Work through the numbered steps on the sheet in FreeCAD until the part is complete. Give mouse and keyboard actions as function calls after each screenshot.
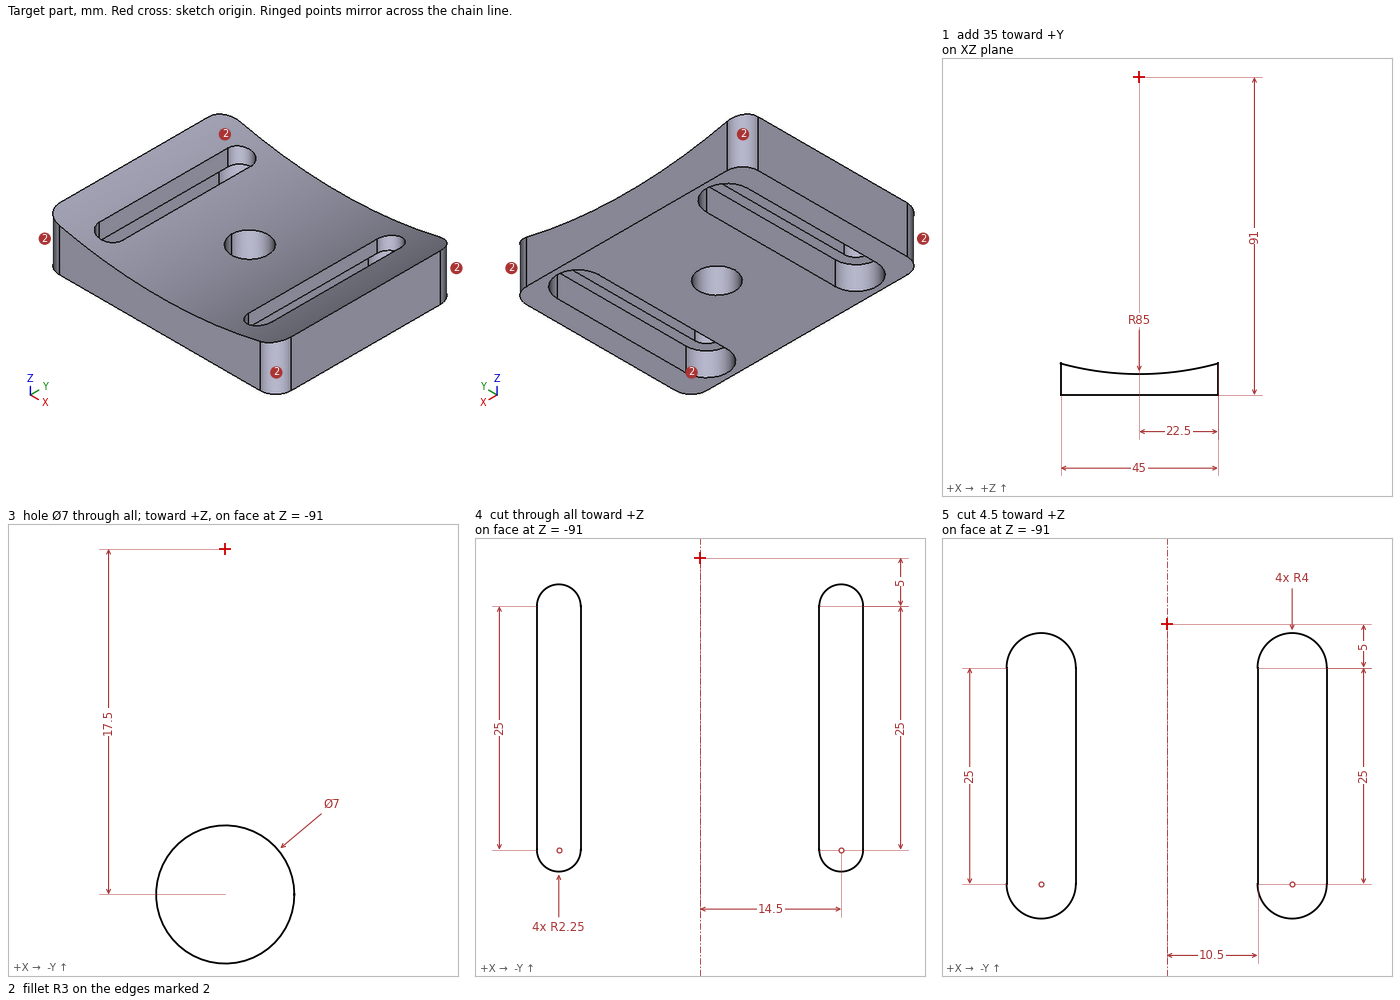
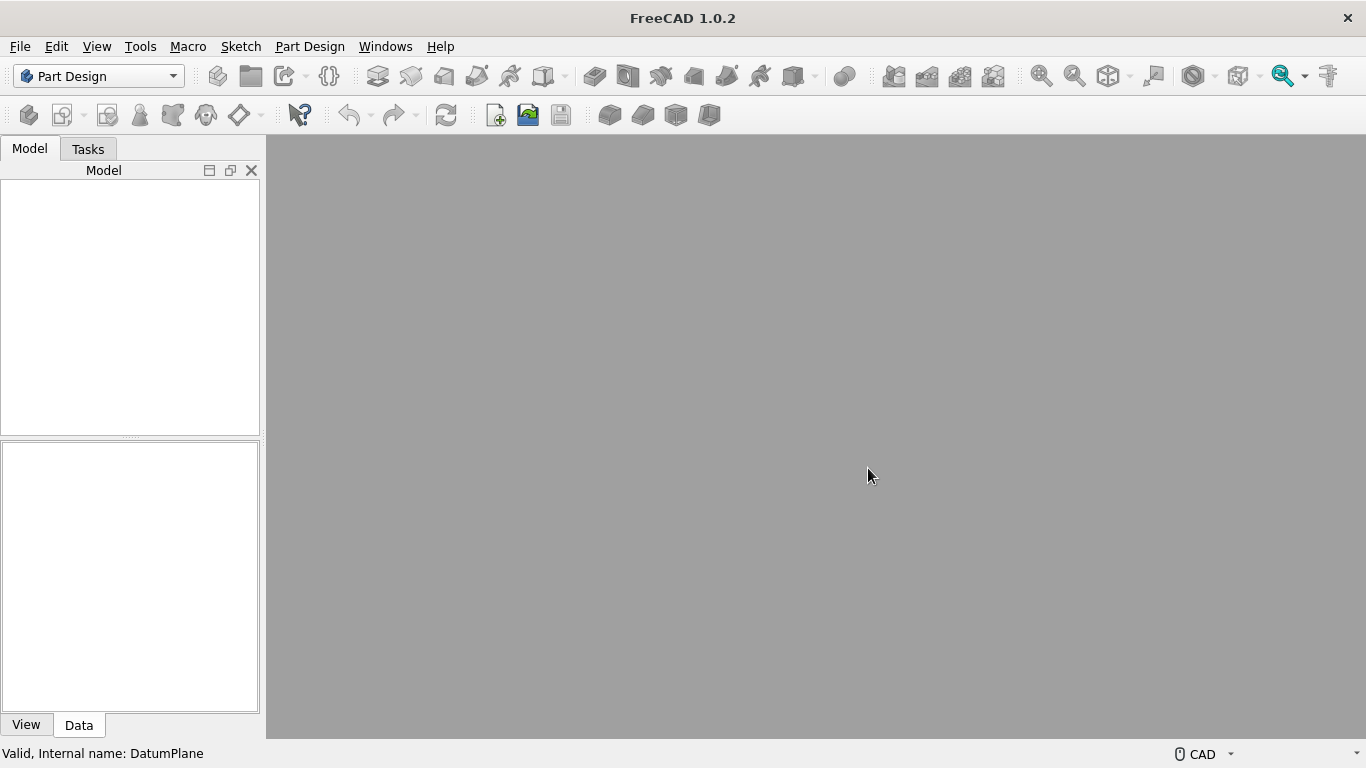
click(495, 116)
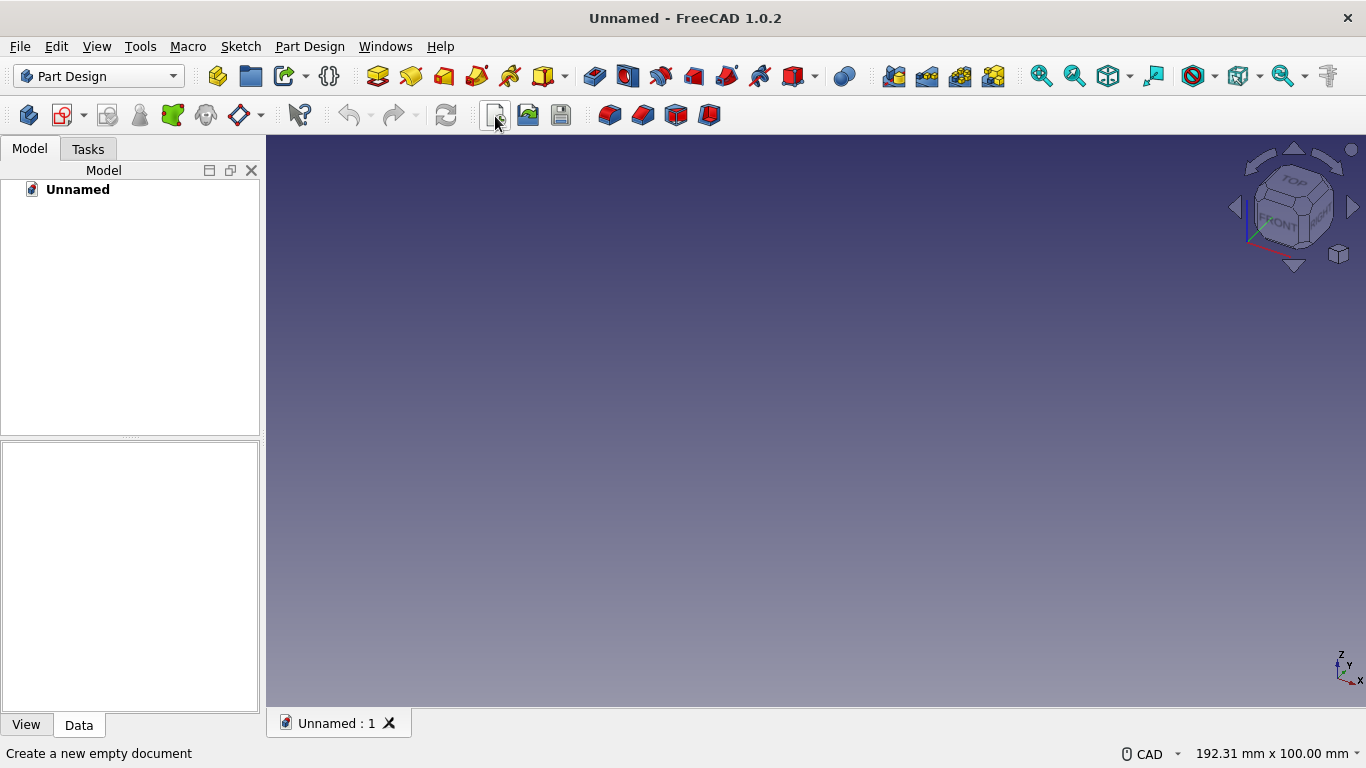
click(62, 116)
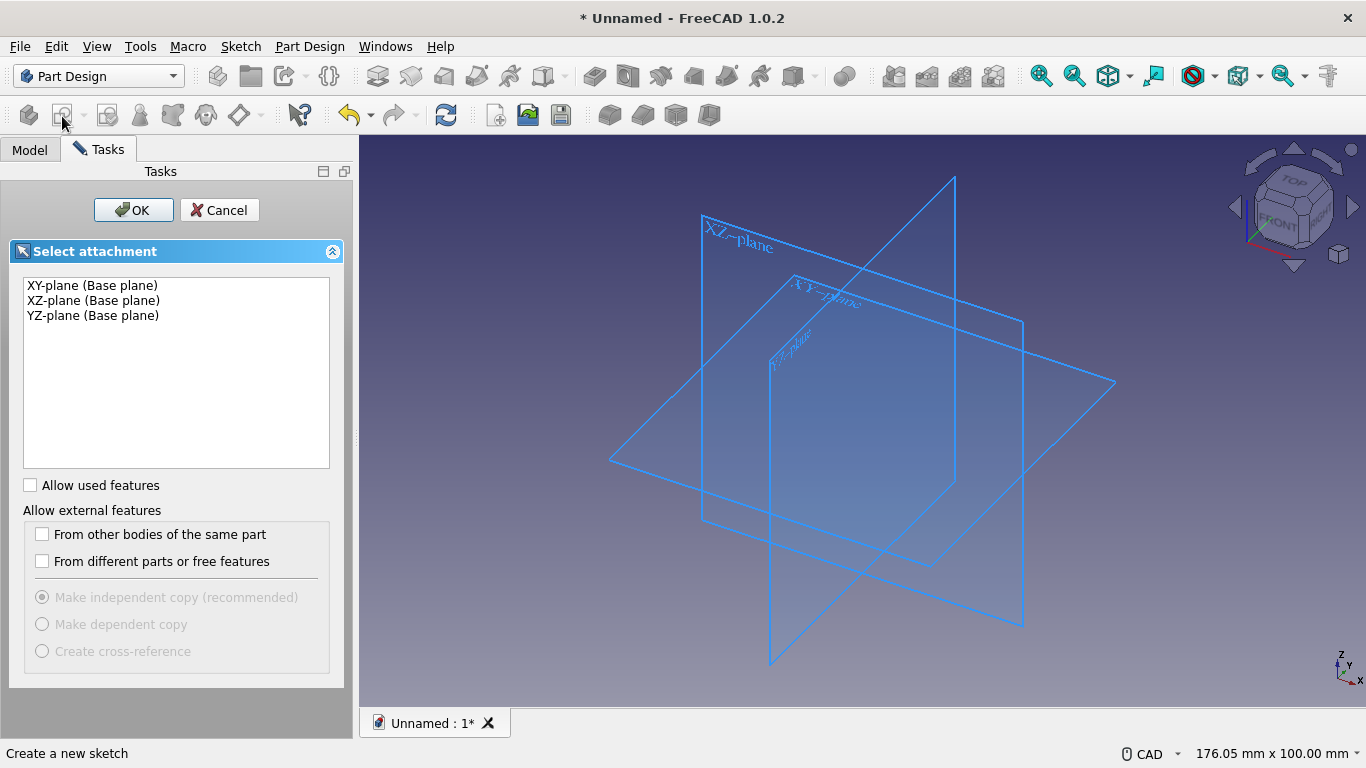
click(84, 300)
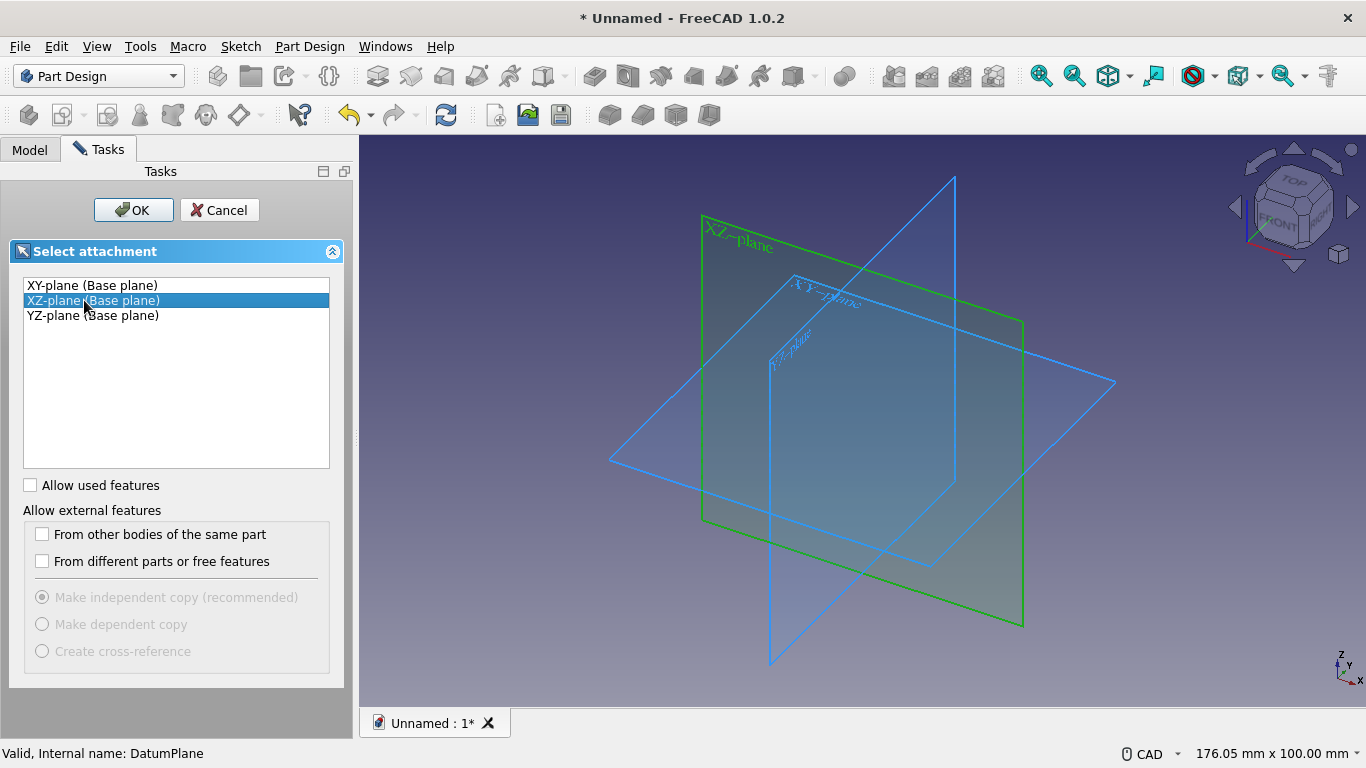
click(134, 210)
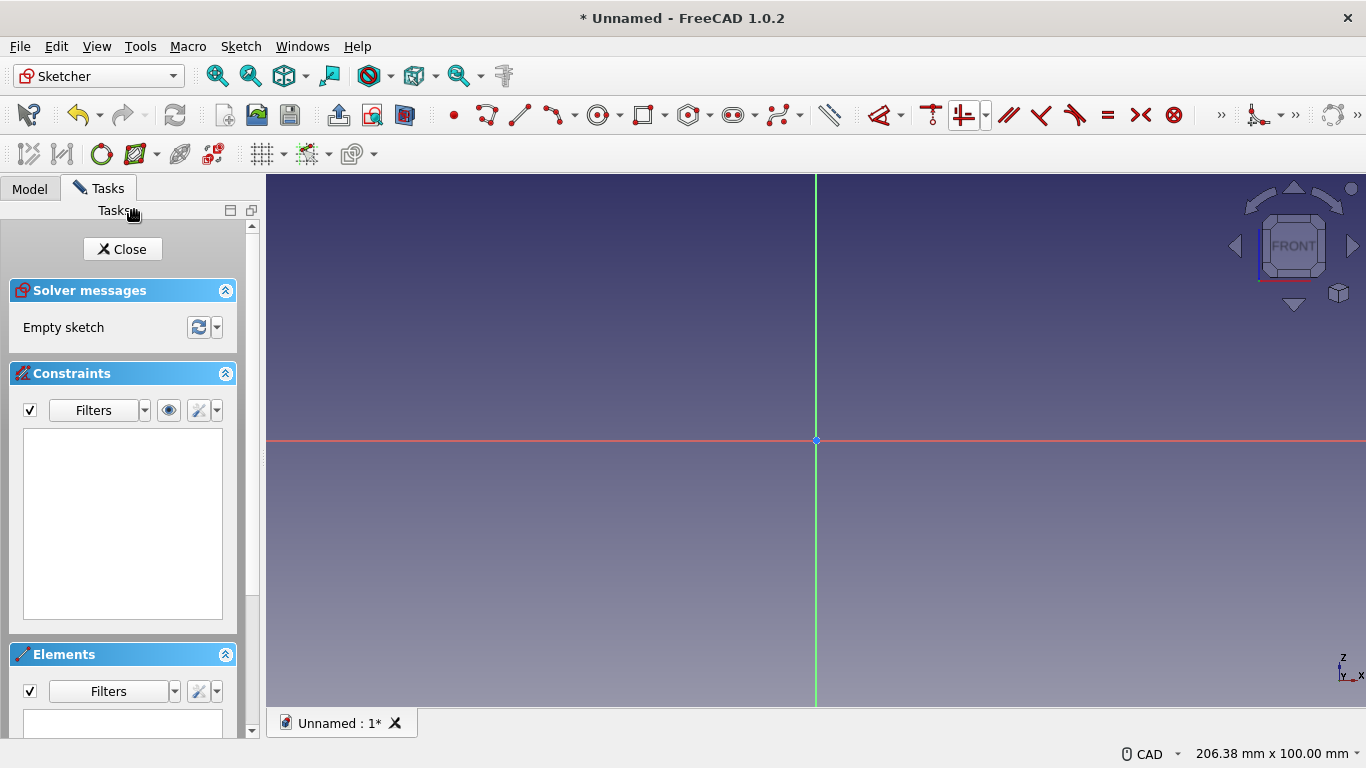
scroll(664, 202, down, 3)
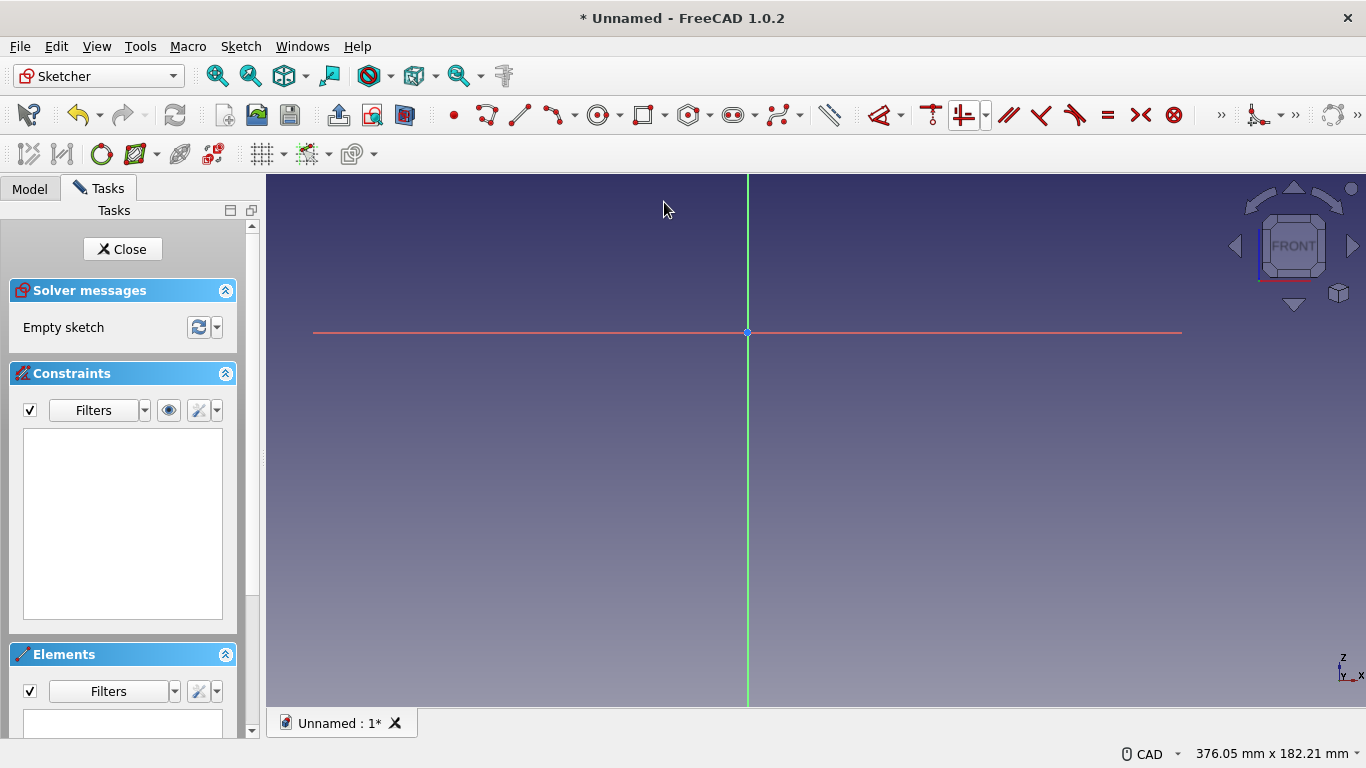
key(g)
key(m)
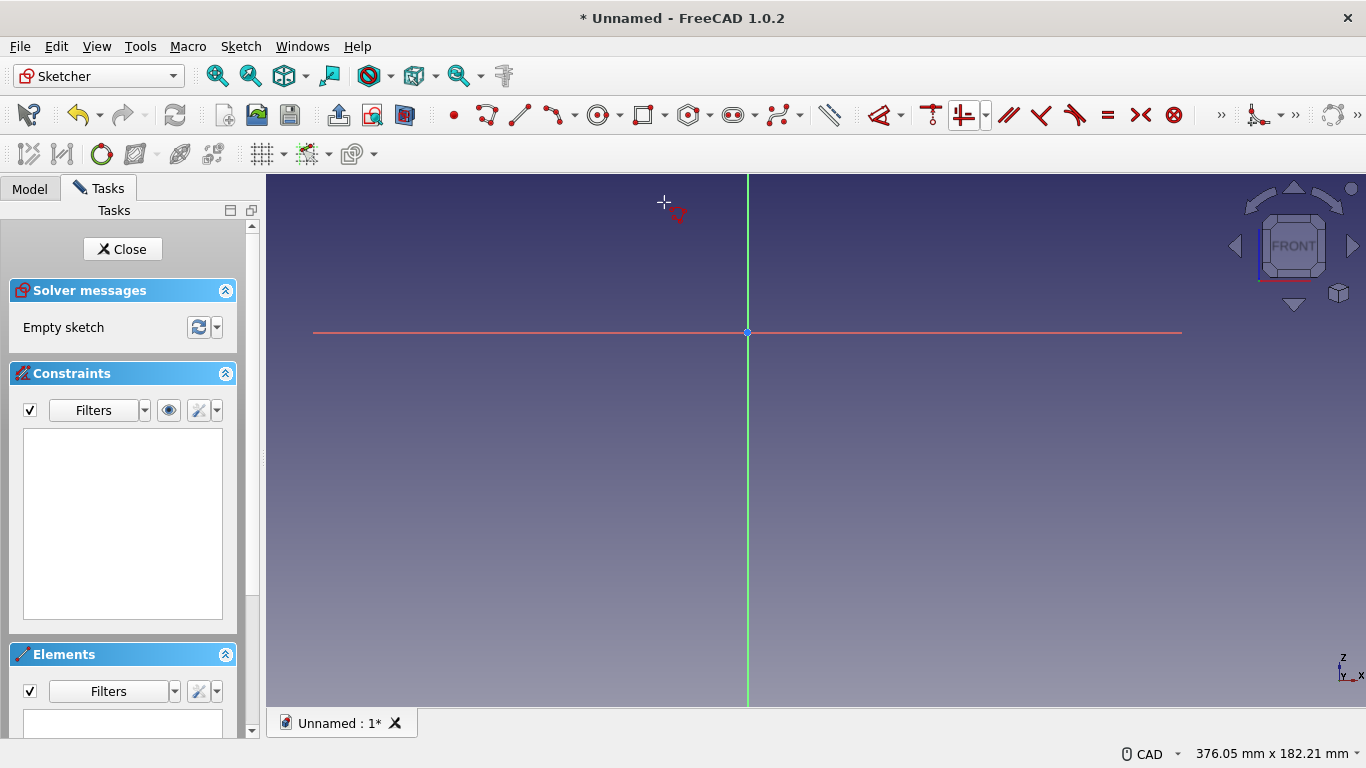
click(813, 573)
click(813, 599)
click(682, 599)
click(682, 573)
right_click(682, 573)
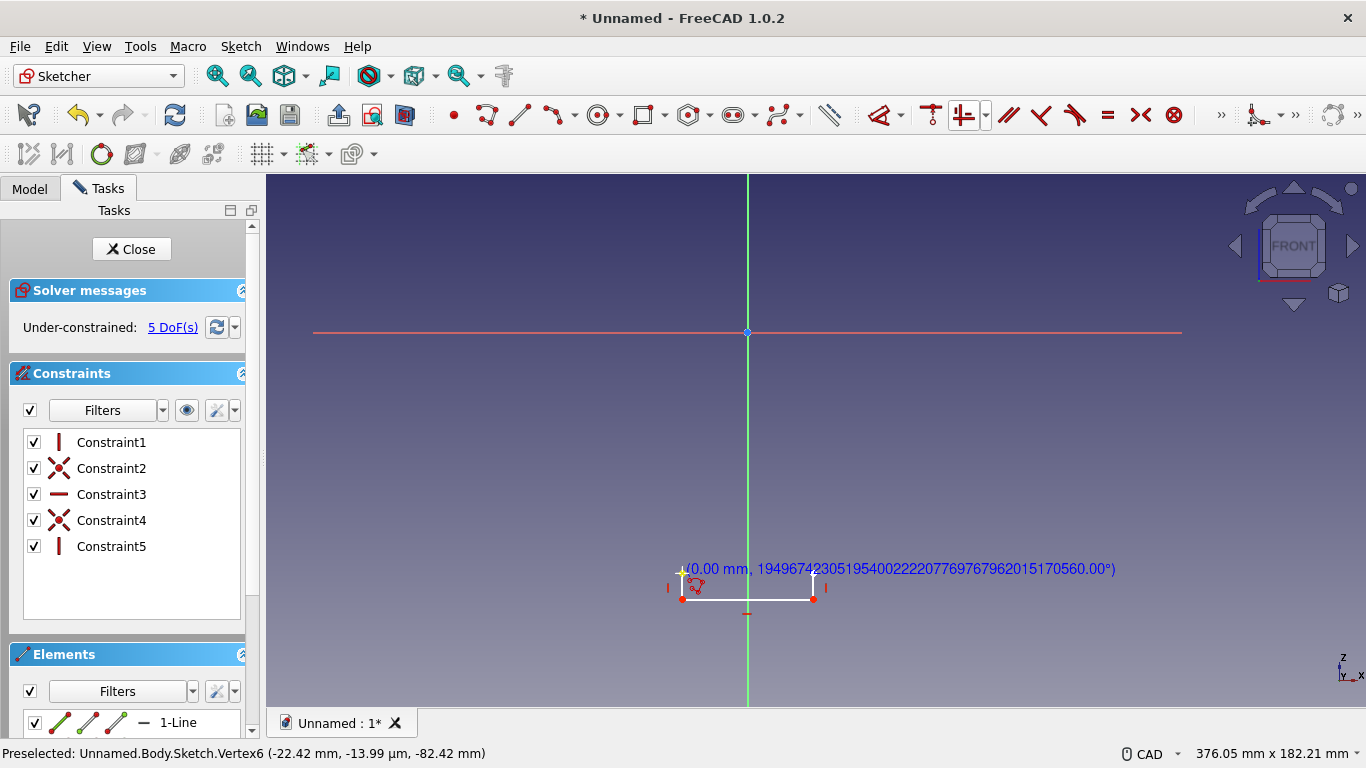
key(g)
key(3)
key(a)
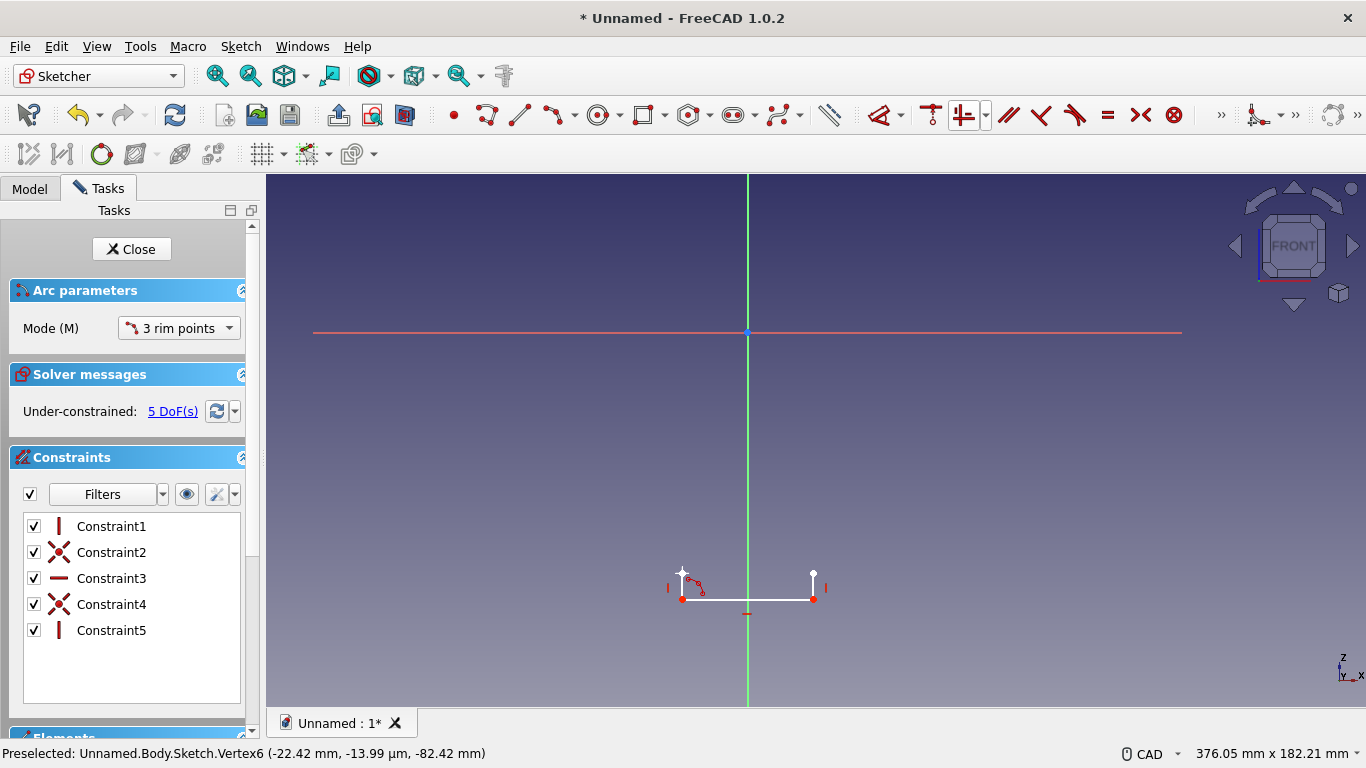
click(682, 574)
click(813, 574)